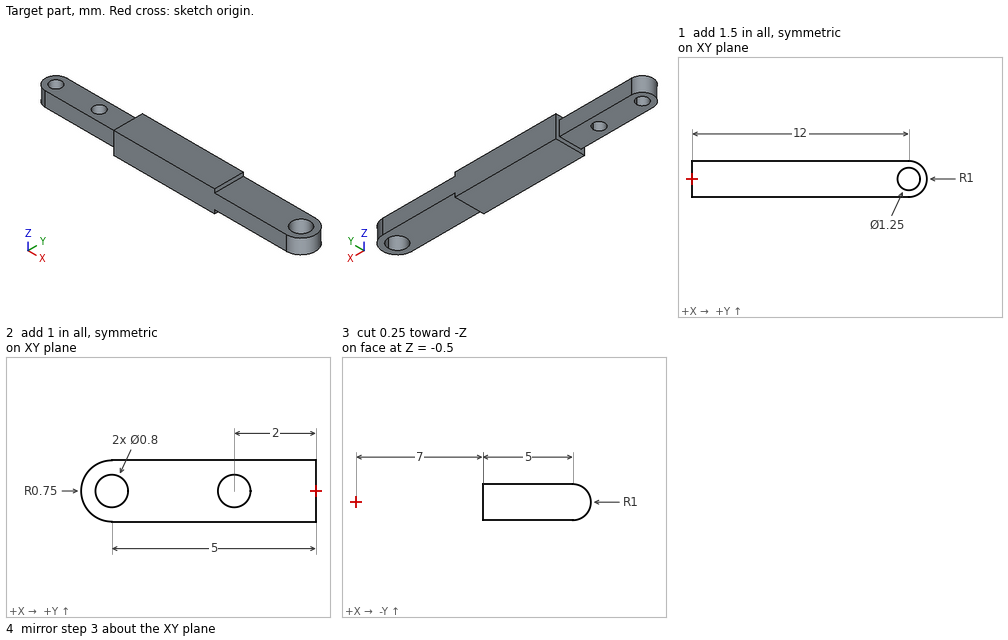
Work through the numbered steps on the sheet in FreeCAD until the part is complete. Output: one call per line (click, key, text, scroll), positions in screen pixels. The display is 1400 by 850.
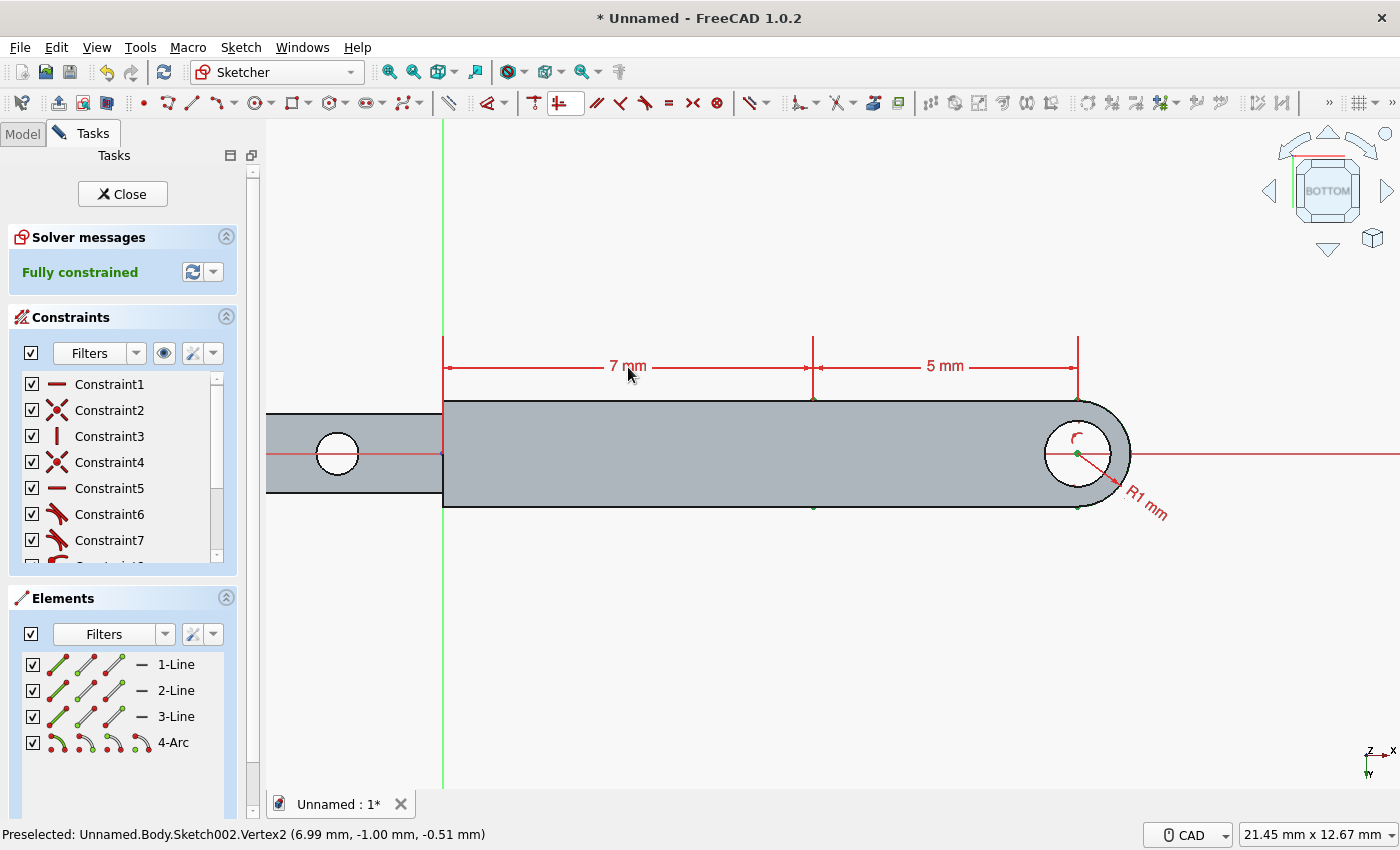
click(123, 194)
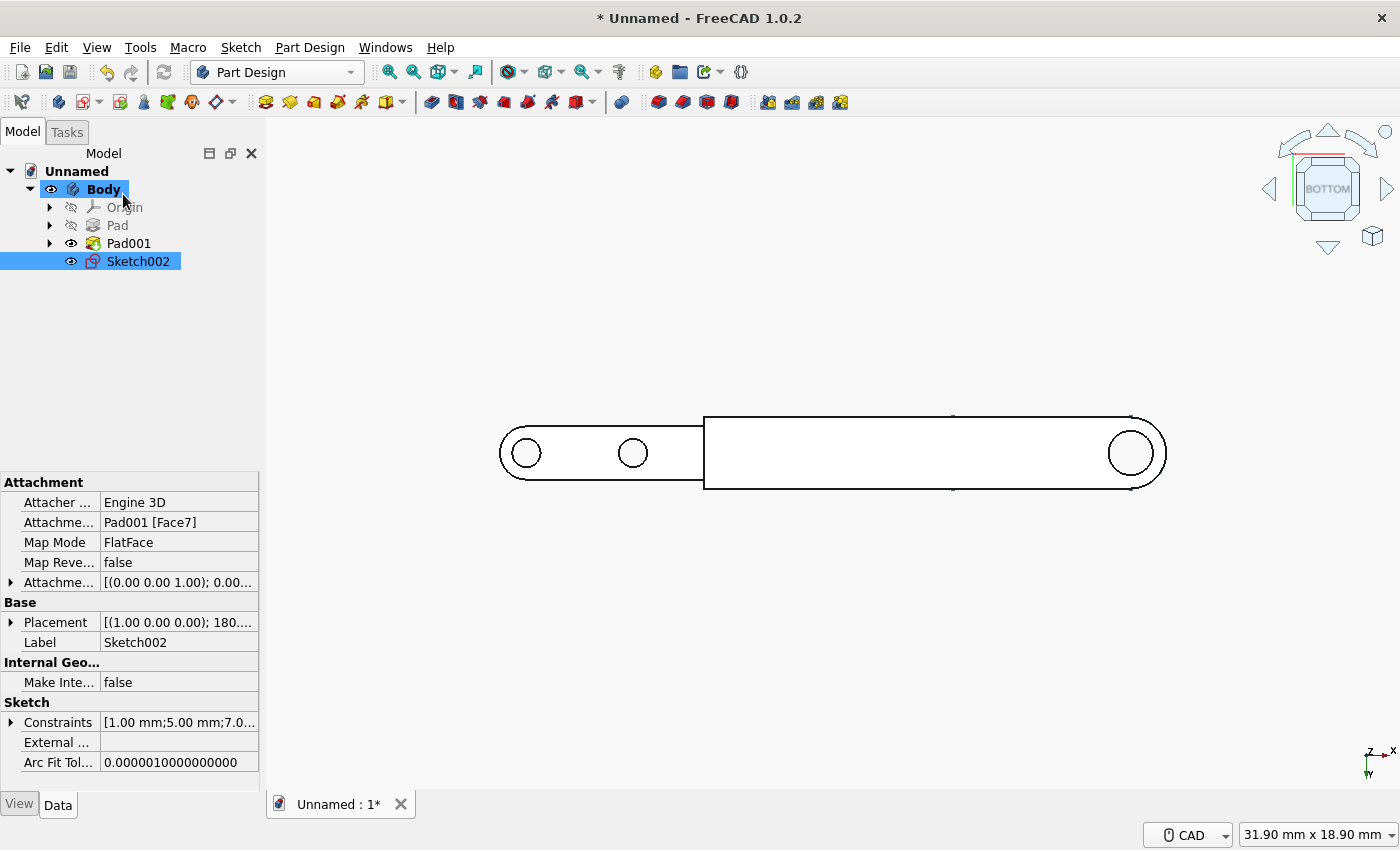
click(432, 102)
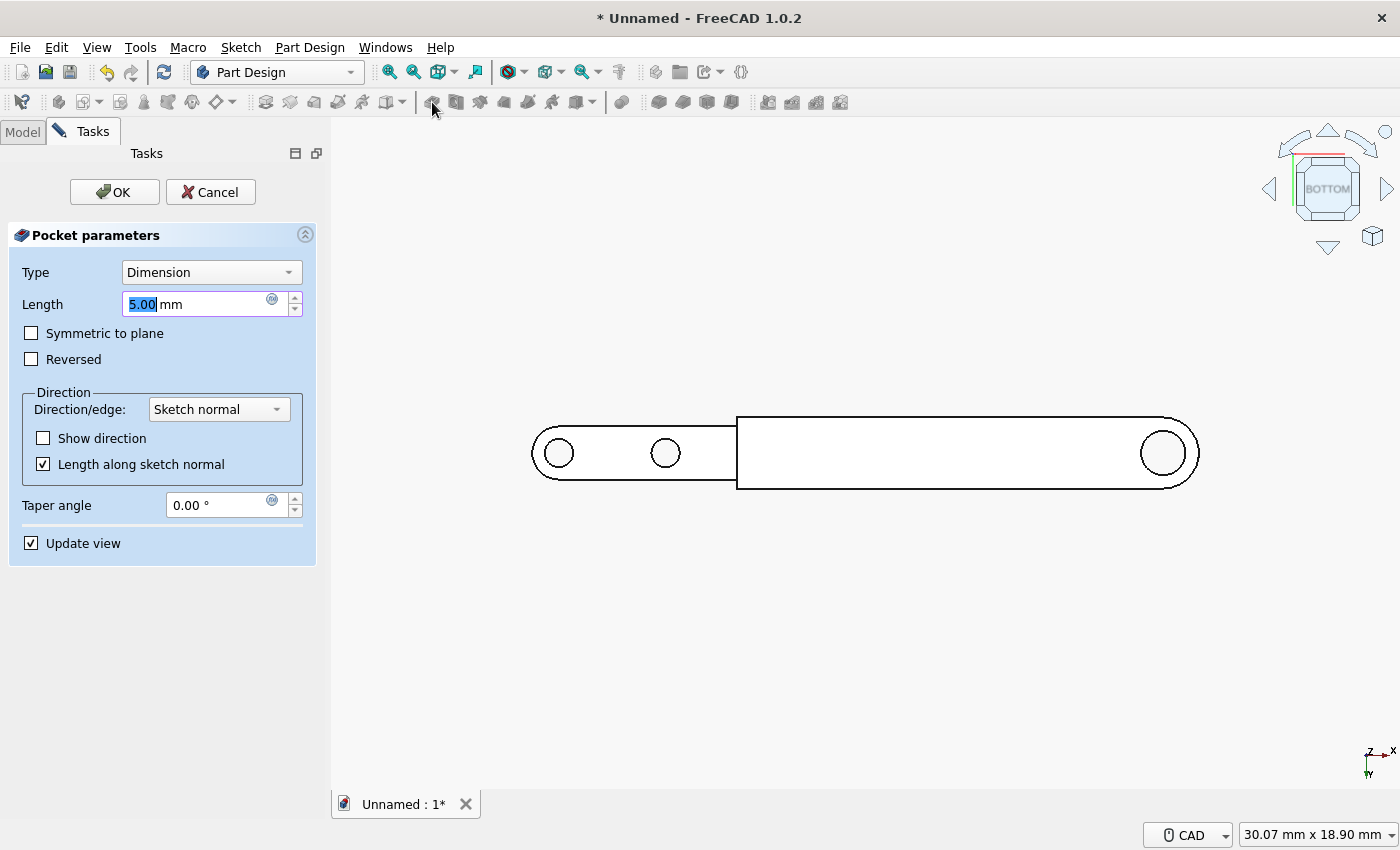
text(0.25)
key(Tab)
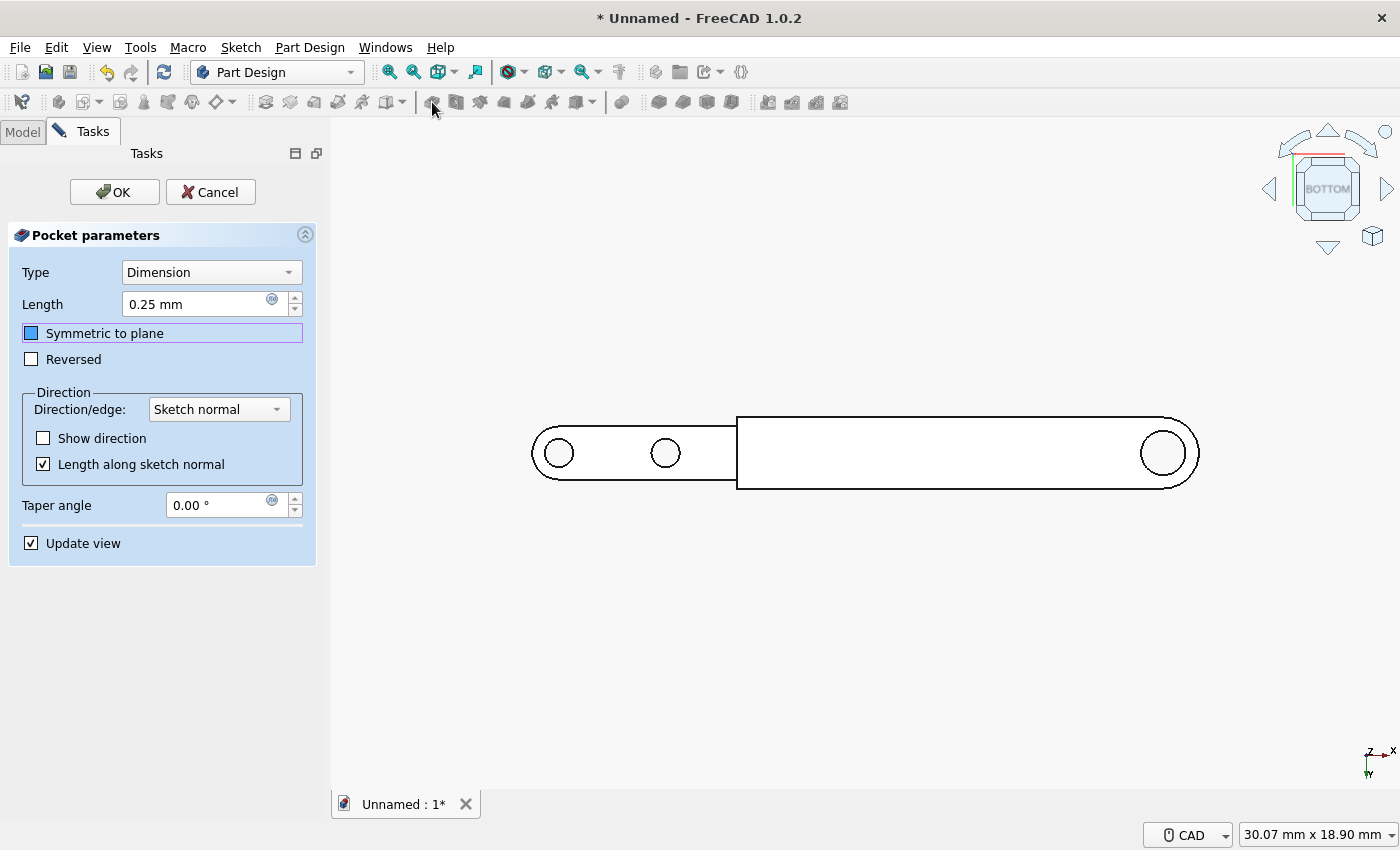
click(30, 359)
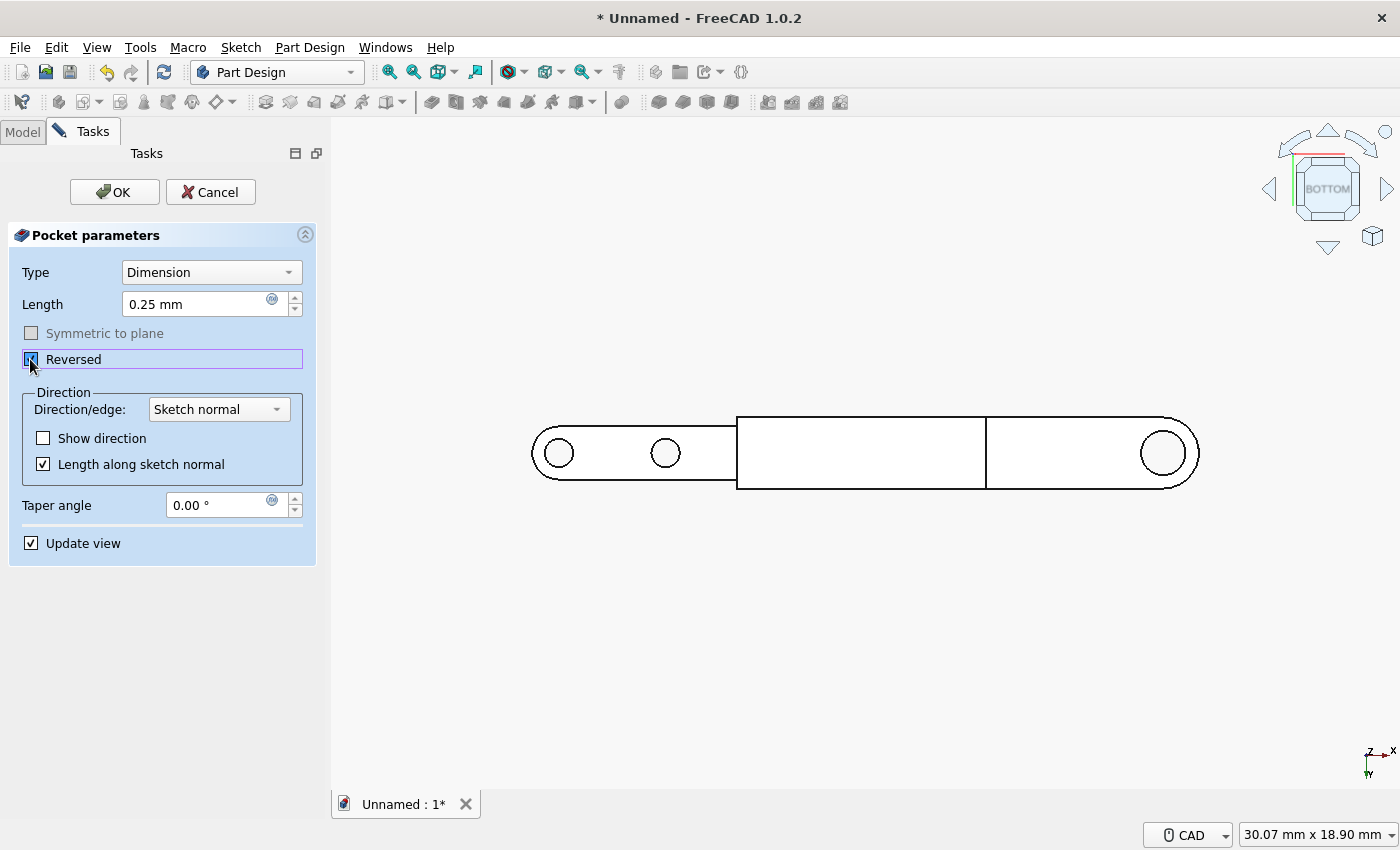
click(115, 192)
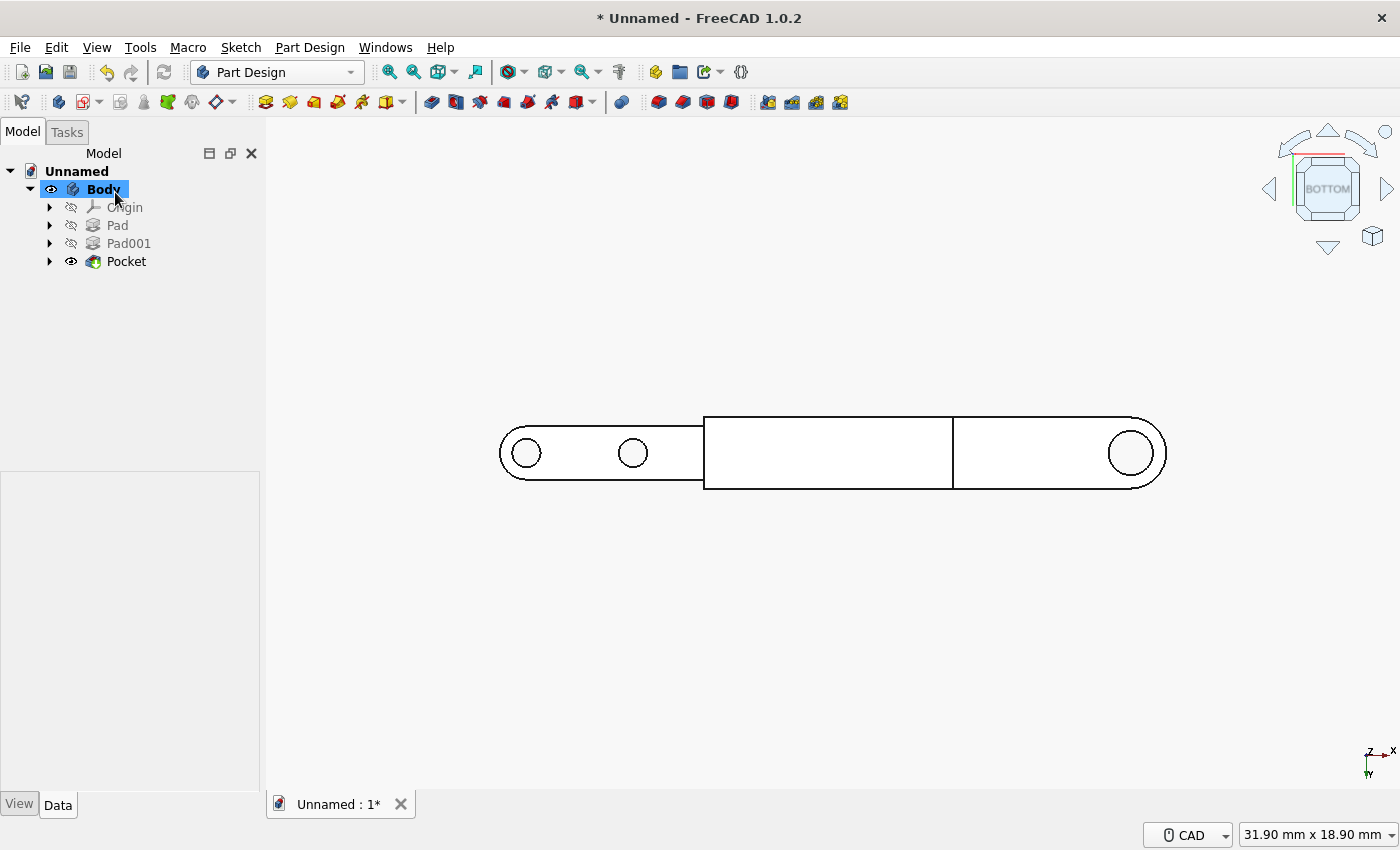
click(116, 261)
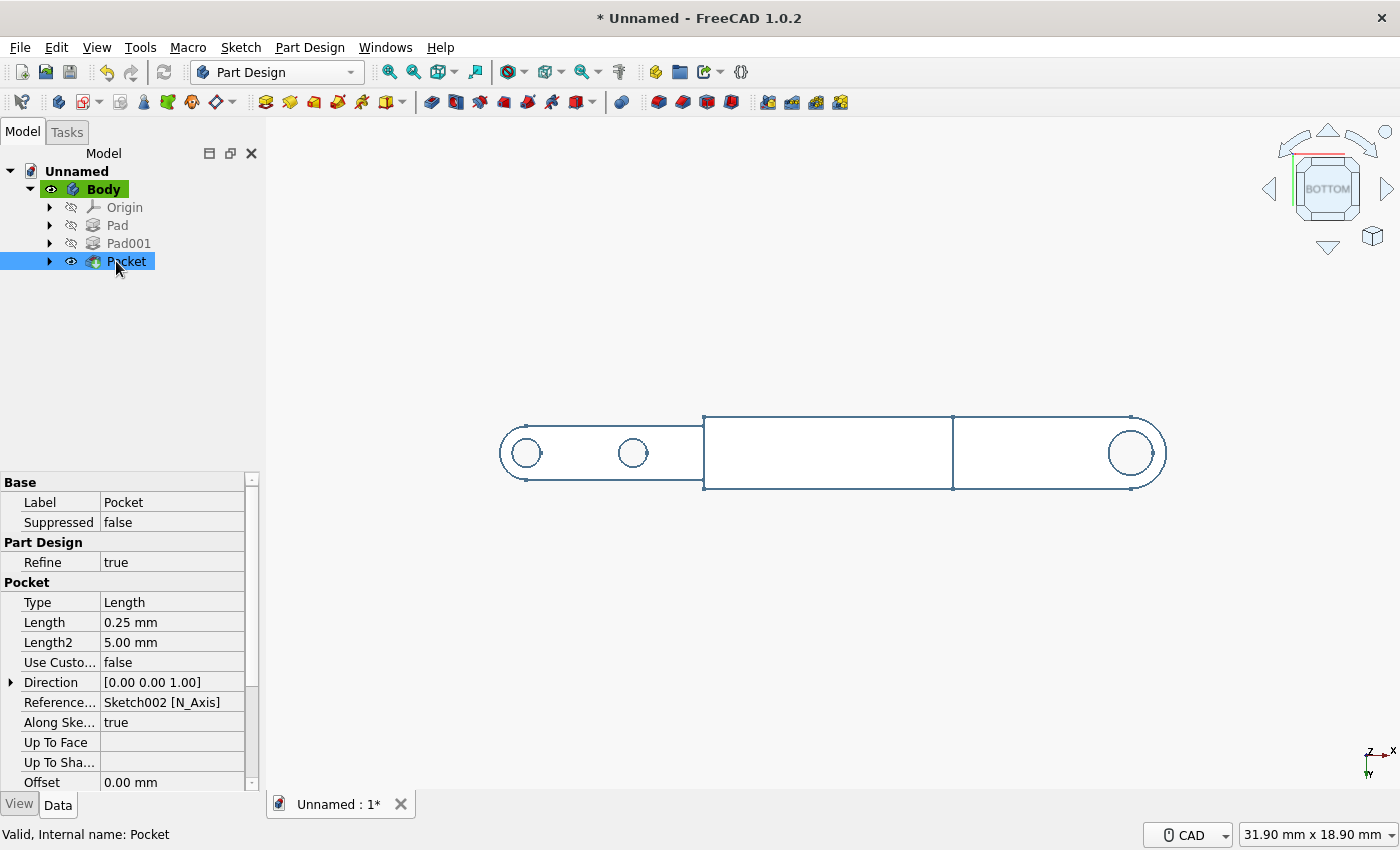
click(768, 102)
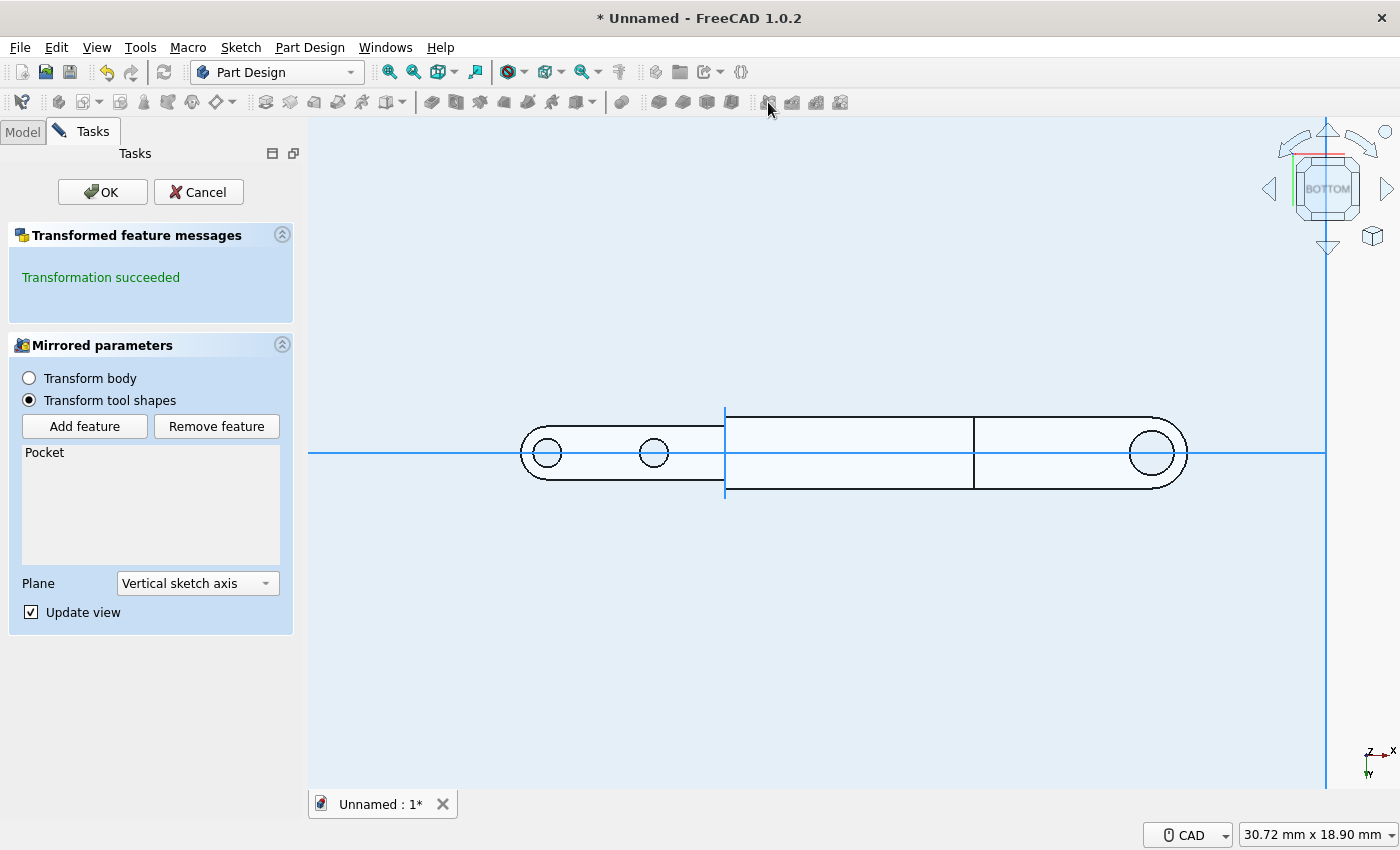
click(198, 584)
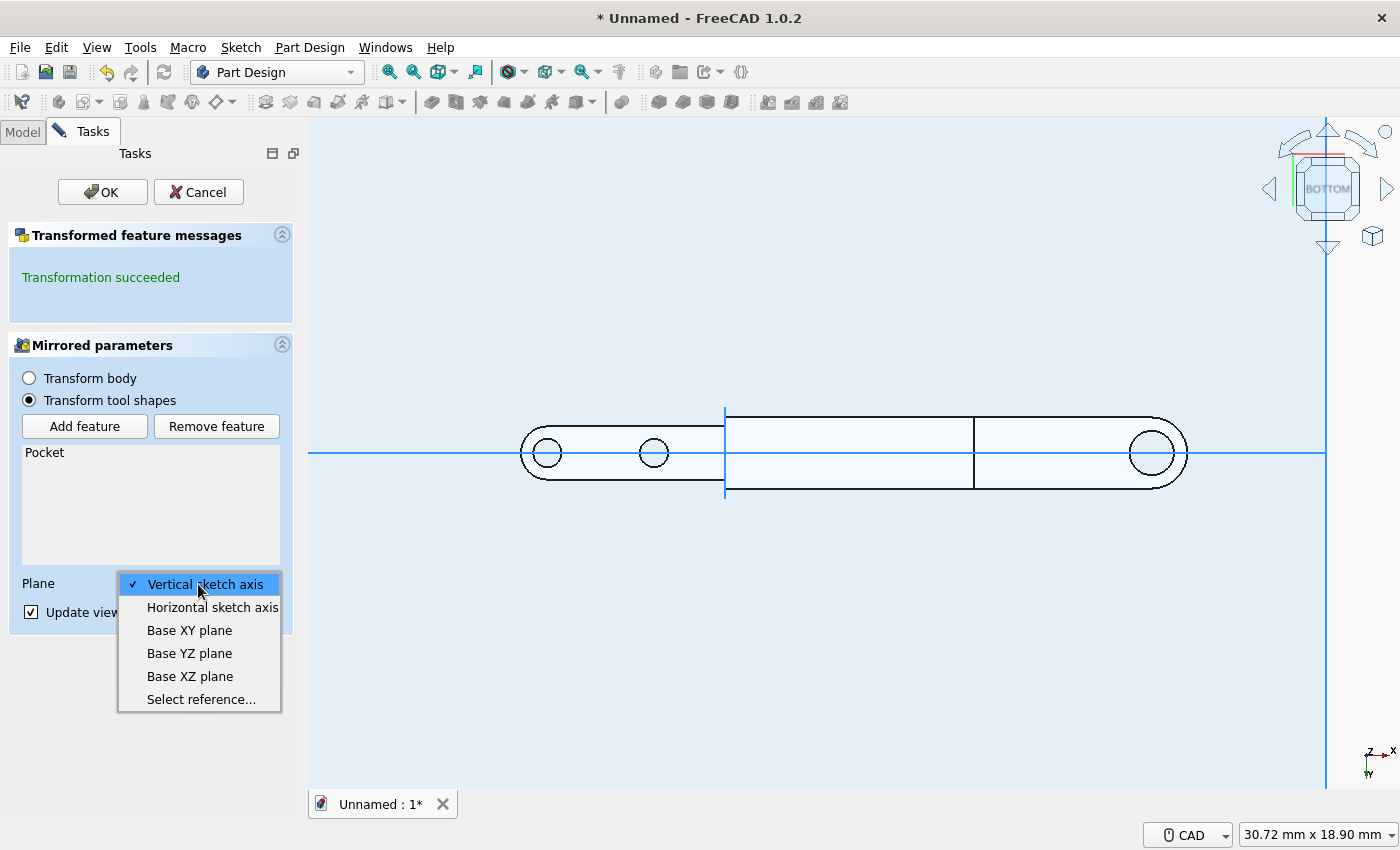
click(198, 630)